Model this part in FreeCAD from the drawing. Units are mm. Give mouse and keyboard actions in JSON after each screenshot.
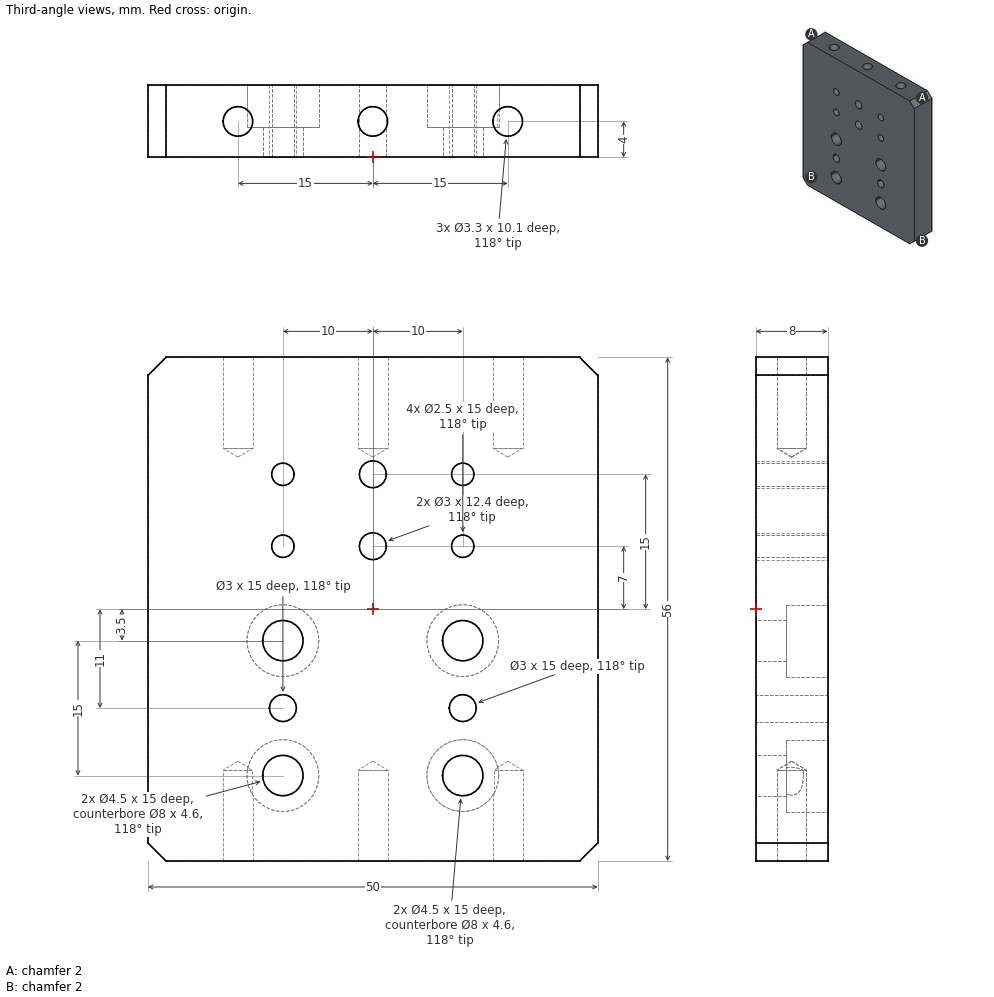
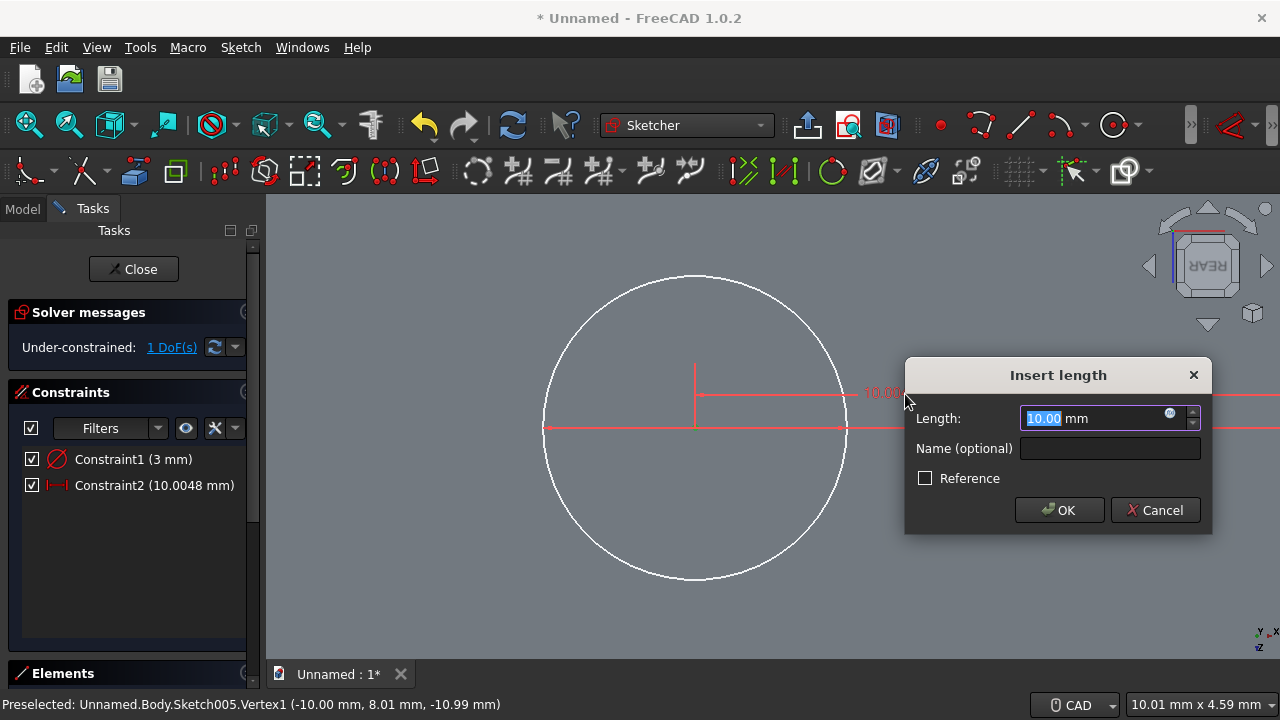
{"action": "type", "text": "10"}
{"action": "key", "text": "Return"}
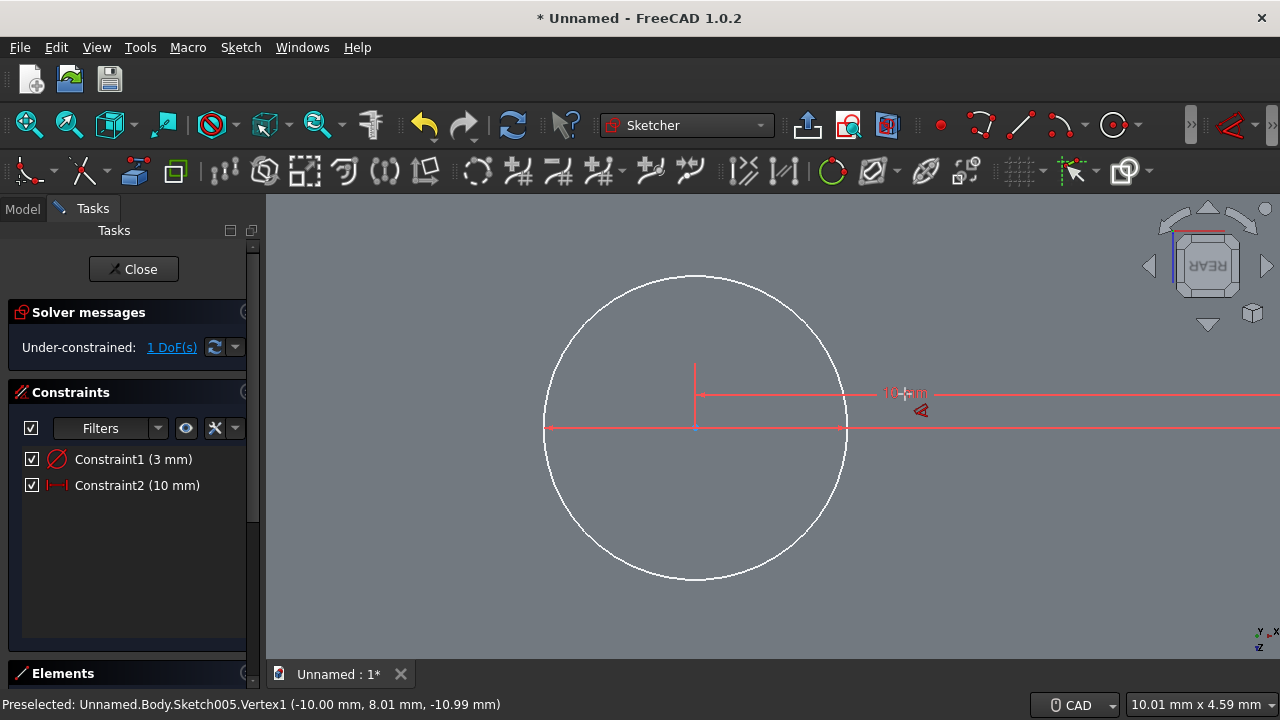
{"action": "left_click", "coordinate": [695, 428]}
{"action": "left_click", "coordinate": [661, 529]}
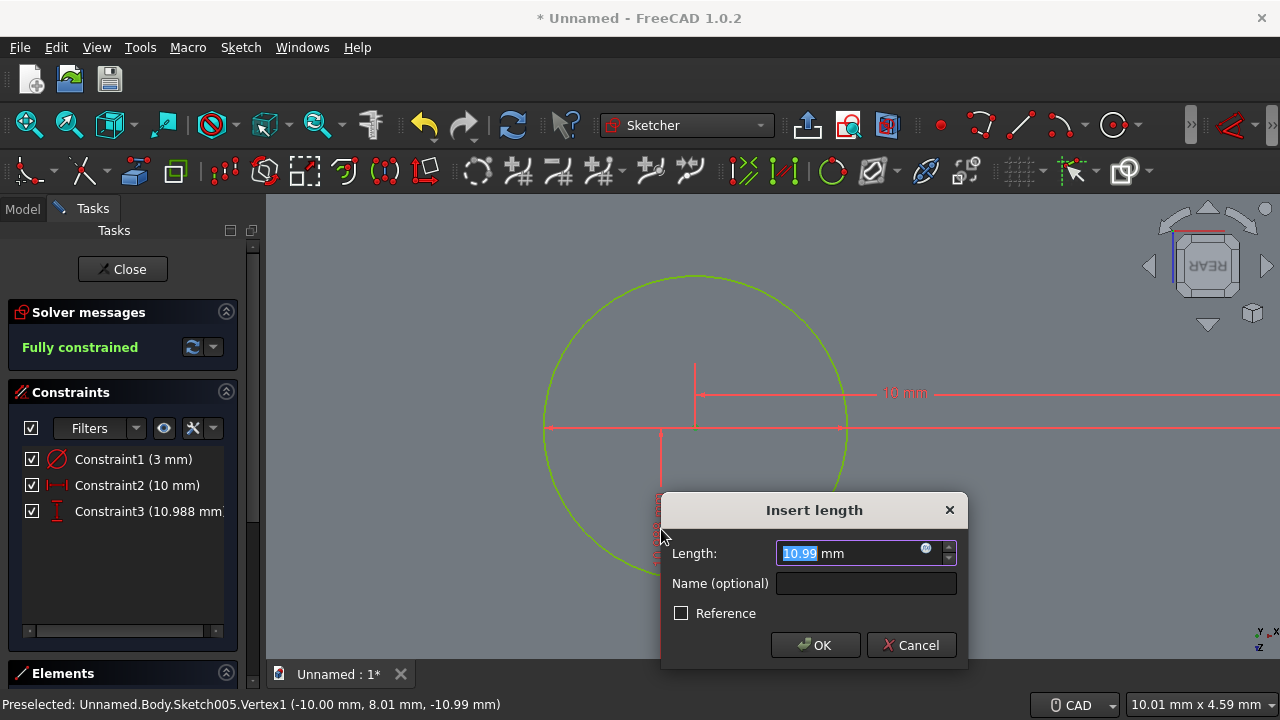
{"action": "type", "text": "11"}
{"action": "key", "text": "Return"}
{"action": "key", "text": "Escape"}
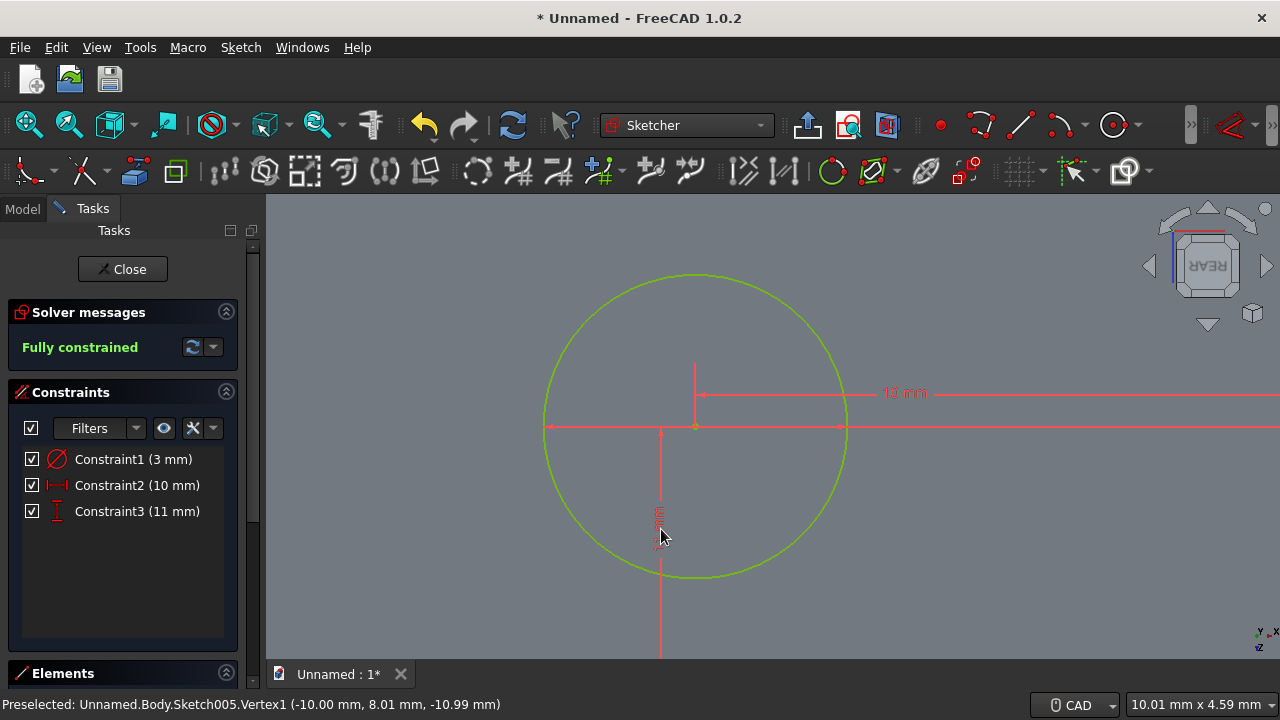
{"action": "left_click", "coordinate": [123, 269]}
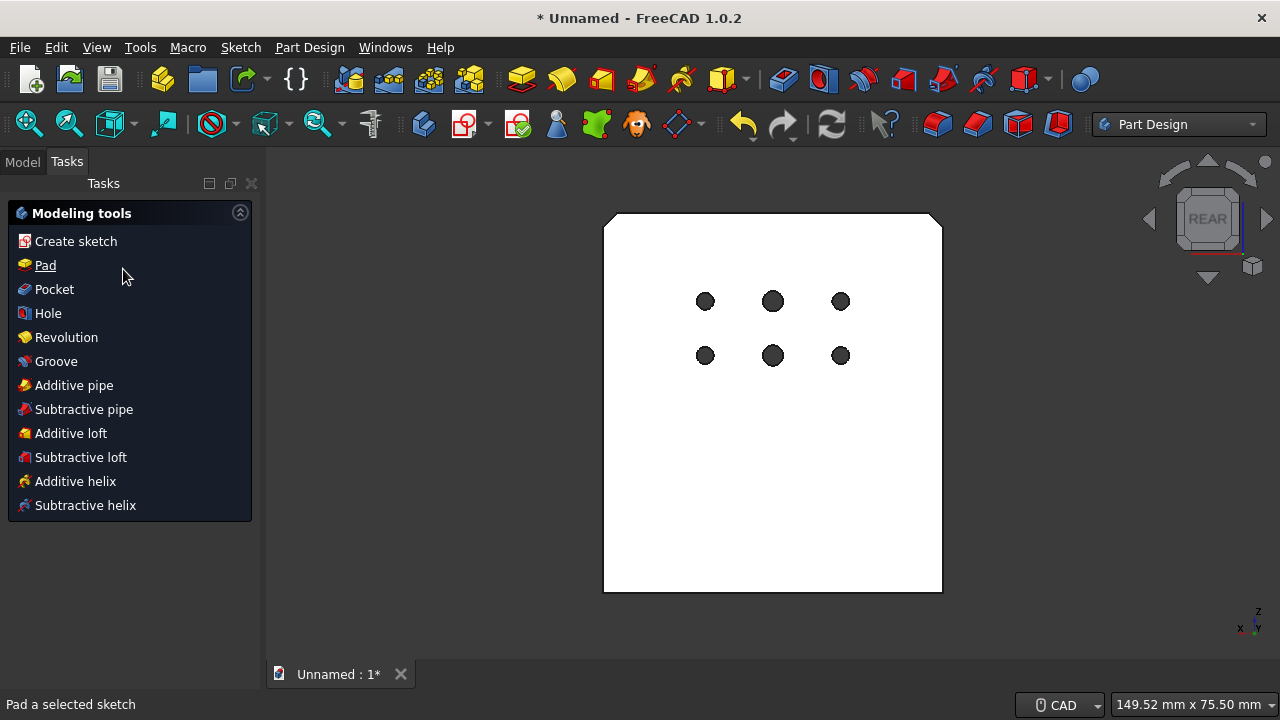
{"action": "left_click", "coordinate": [824, 80]}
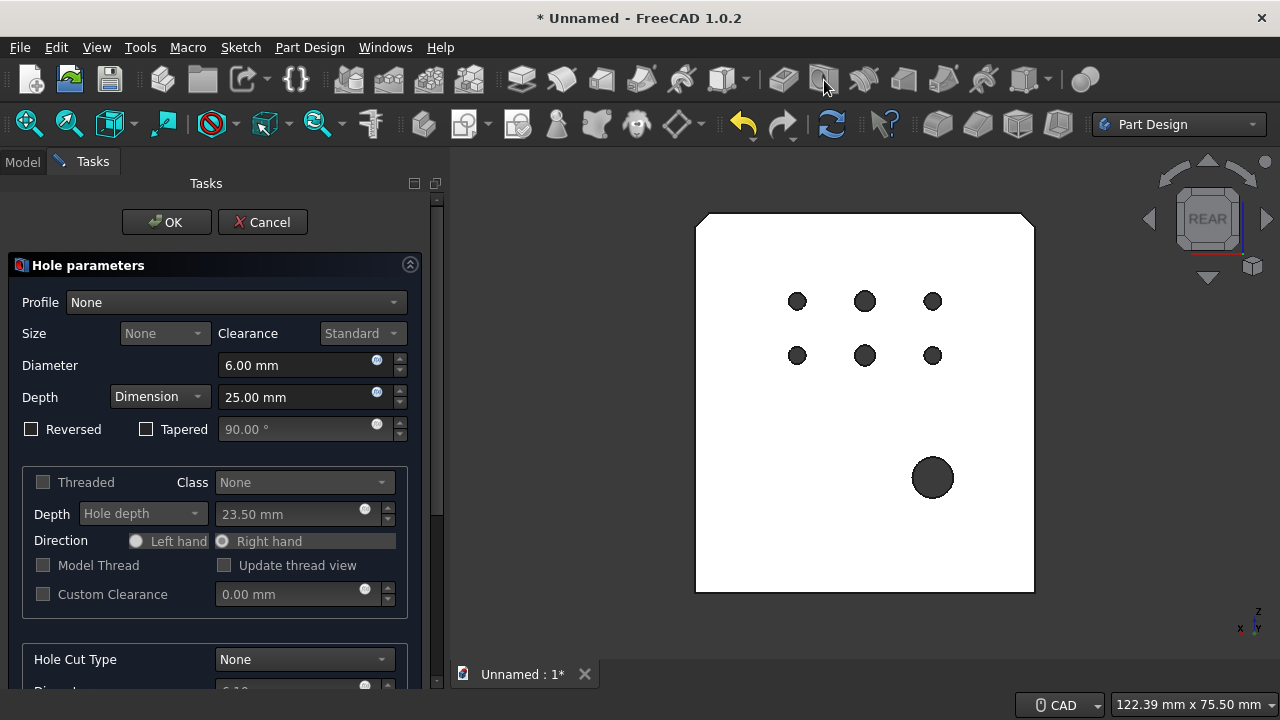
{"action": "triple_click", "coordinate": [305, 365]}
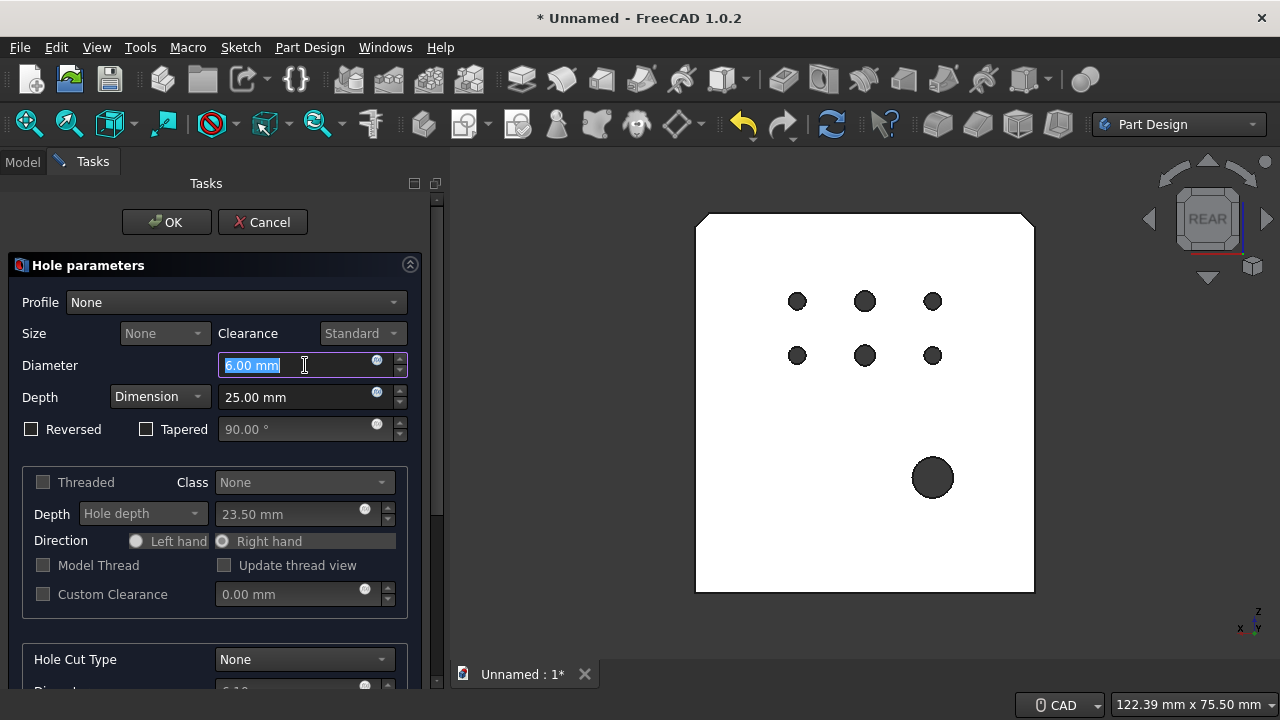
{"action": "type", "text": "3"}
{"action": "key", "text": "Tab"}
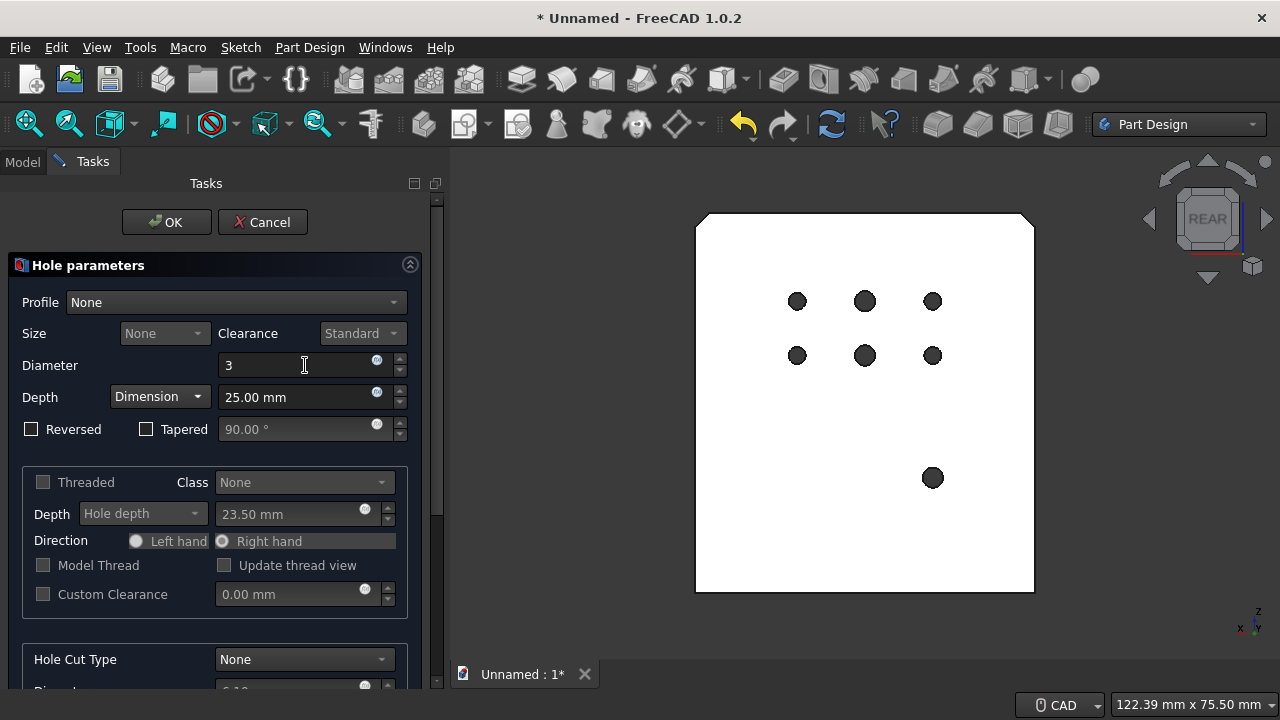
{"action": "triple_click", "coordinate": [305, 397]}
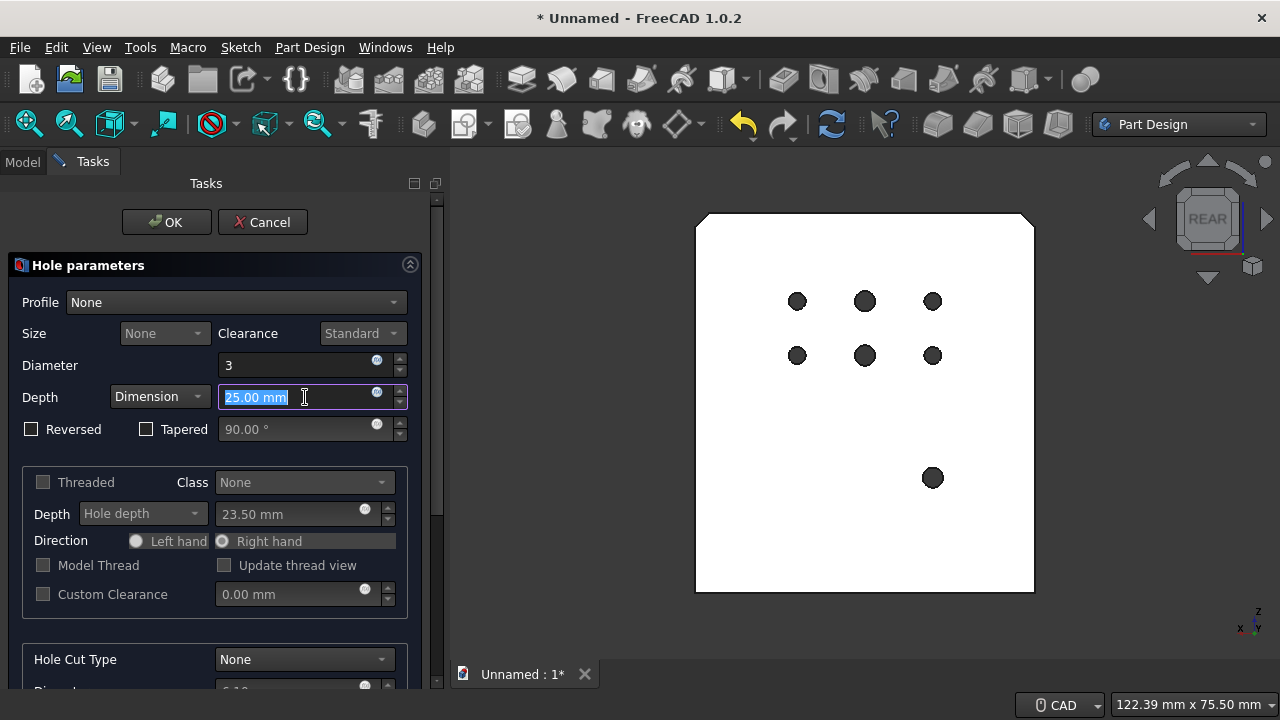
{"action": "type", "text": "15"}
{"action": "key", "text": "Tab"}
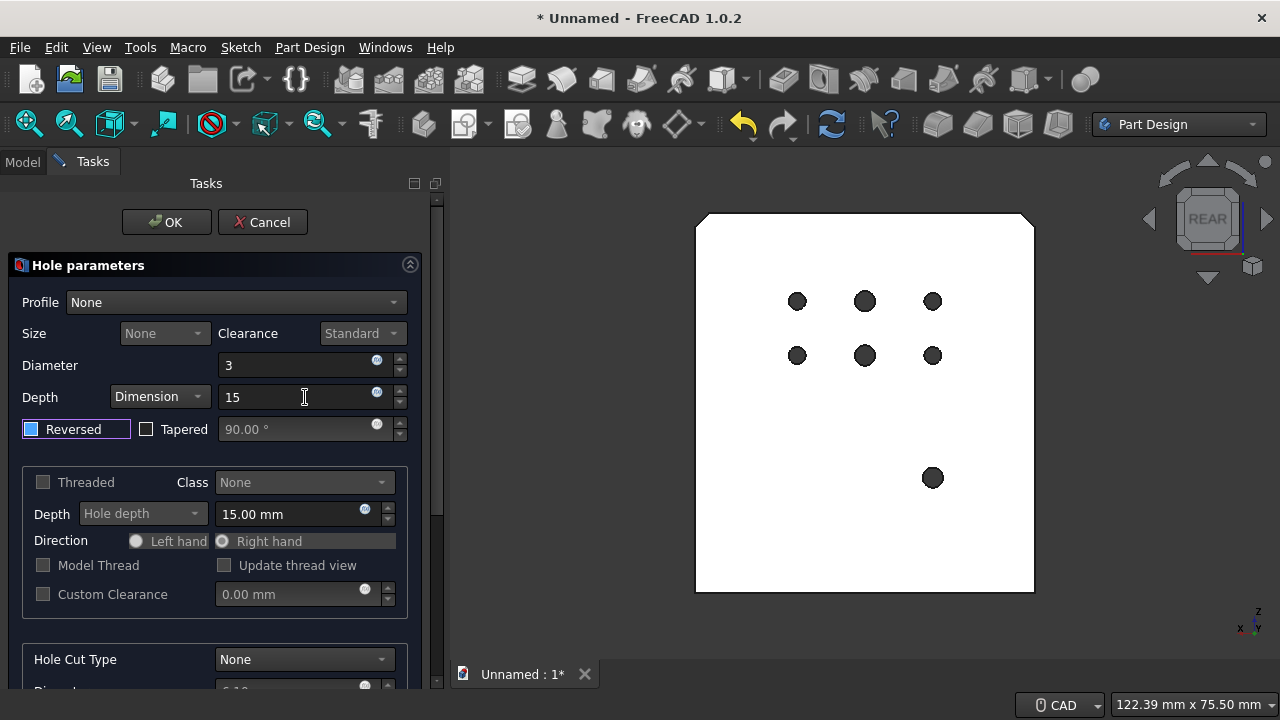
{"action": "left_click", "coordinate": [167, 222]}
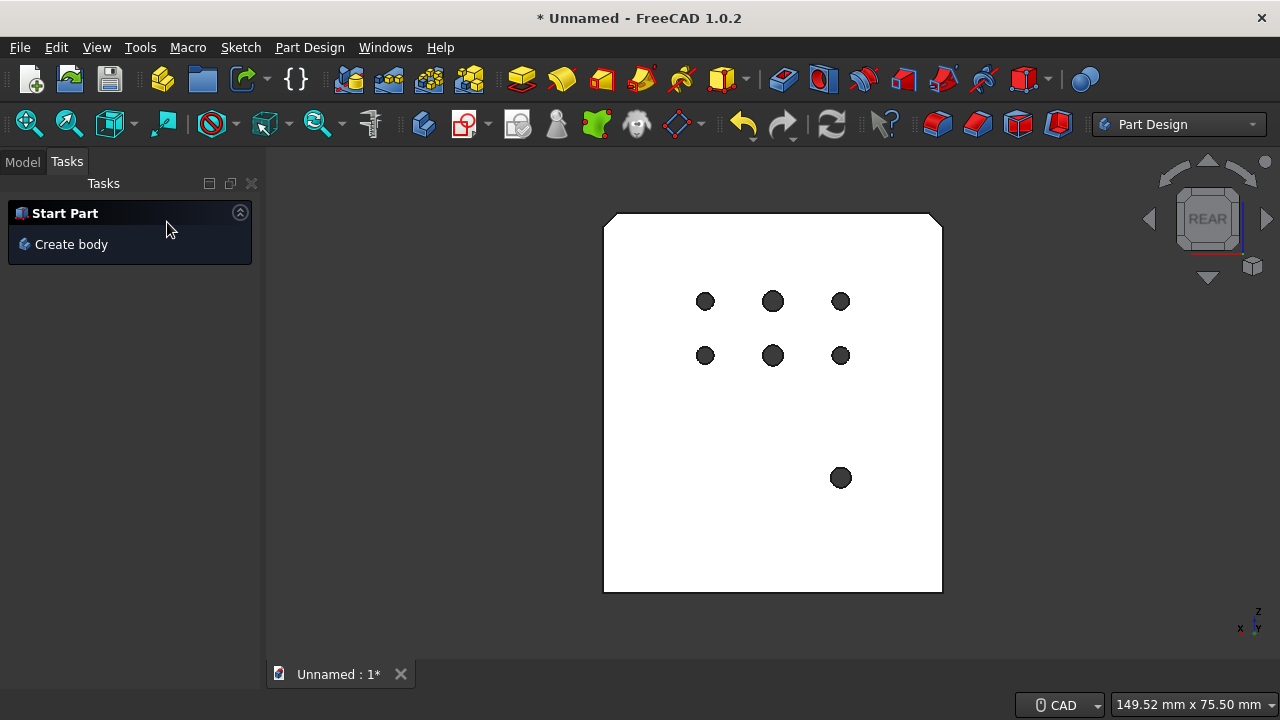
{"action": "left_click", "coordinate": [725, 456]}